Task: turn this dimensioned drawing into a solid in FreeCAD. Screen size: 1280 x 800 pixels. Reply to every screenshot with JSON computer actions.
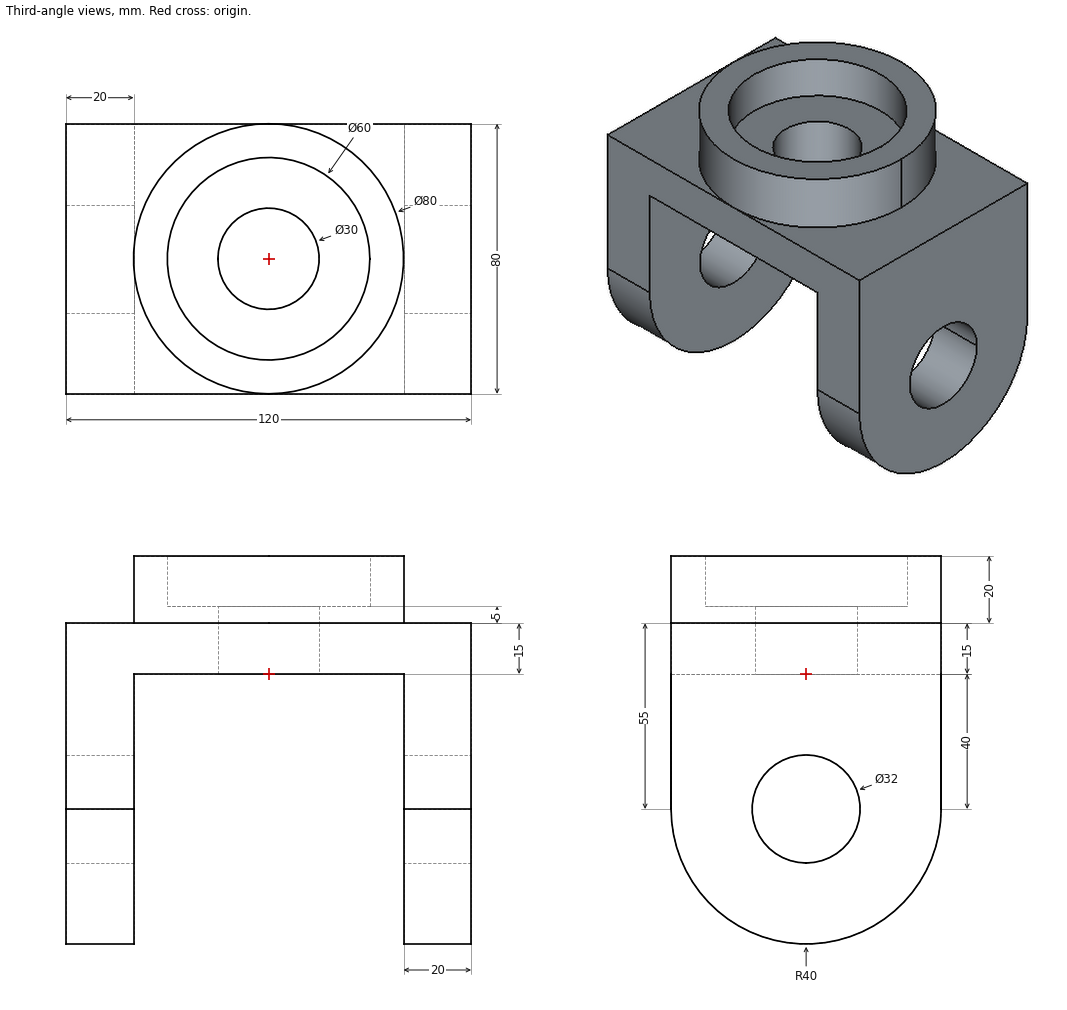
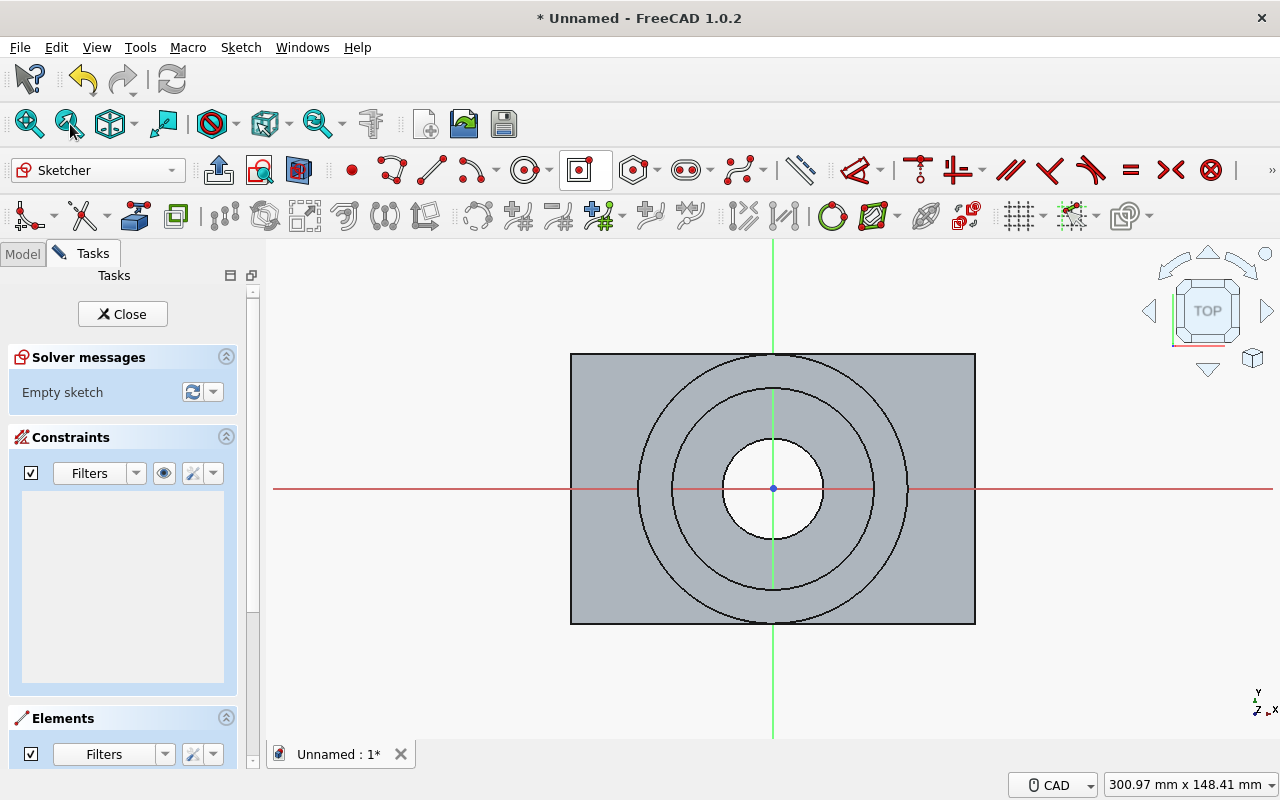
{"action": "left_click", "coordinate": [300, 170]}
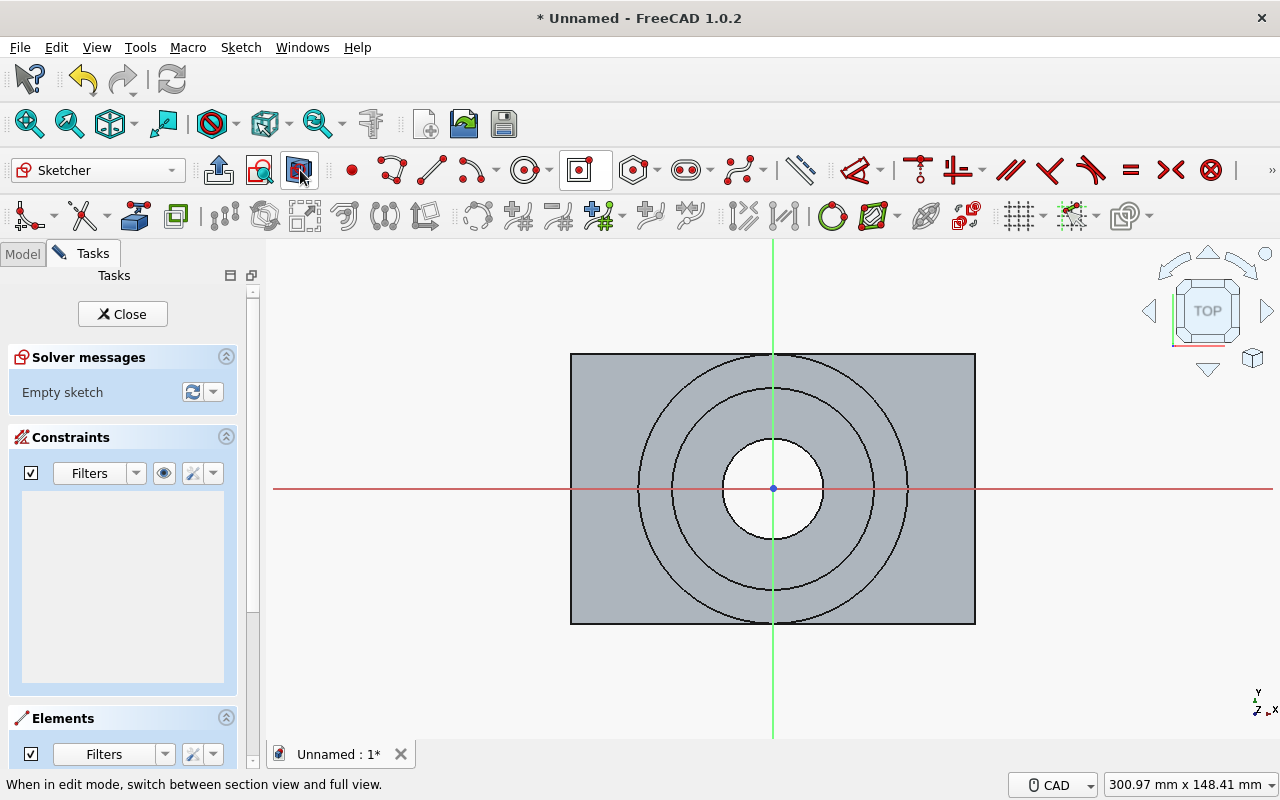
{"action": "scroll", "coordinate": [912, 489], "scroll_direction": "up", "scroll_amount": 2}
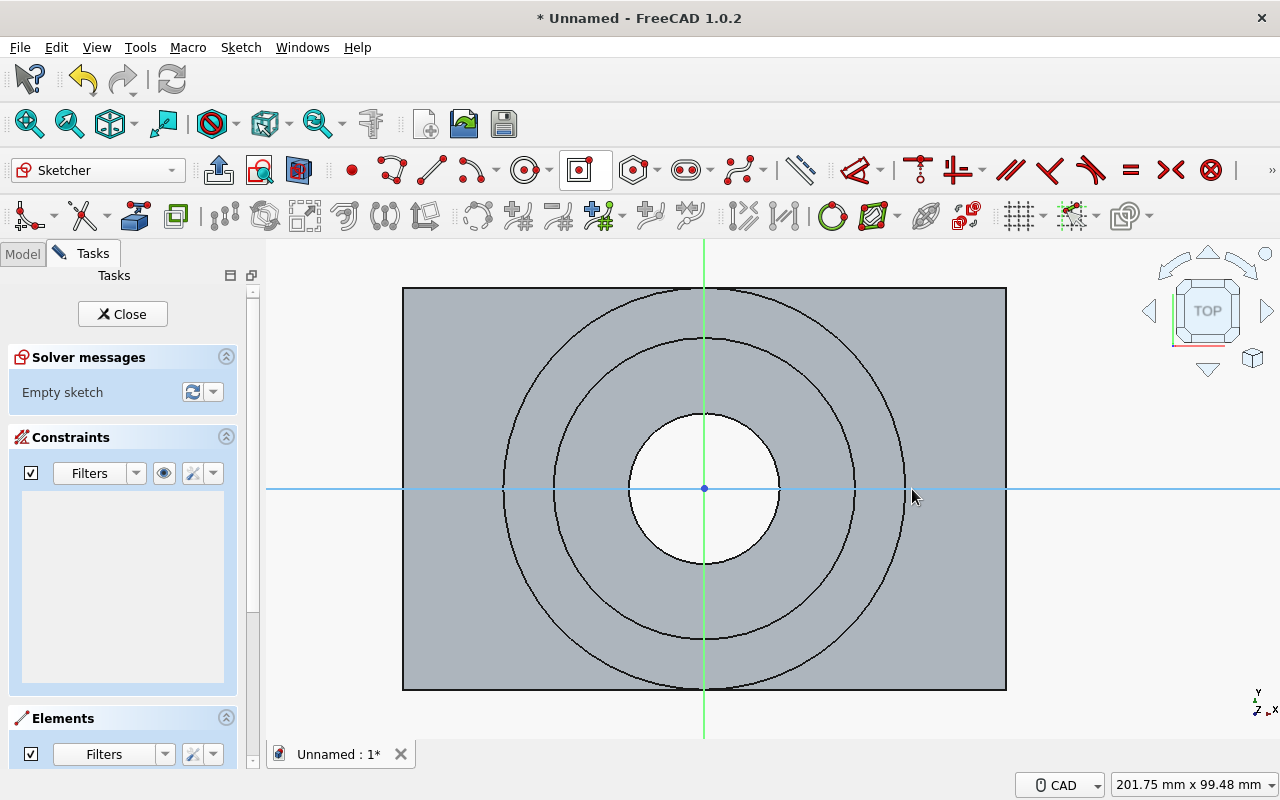
{"action": "key", "text": "g c"}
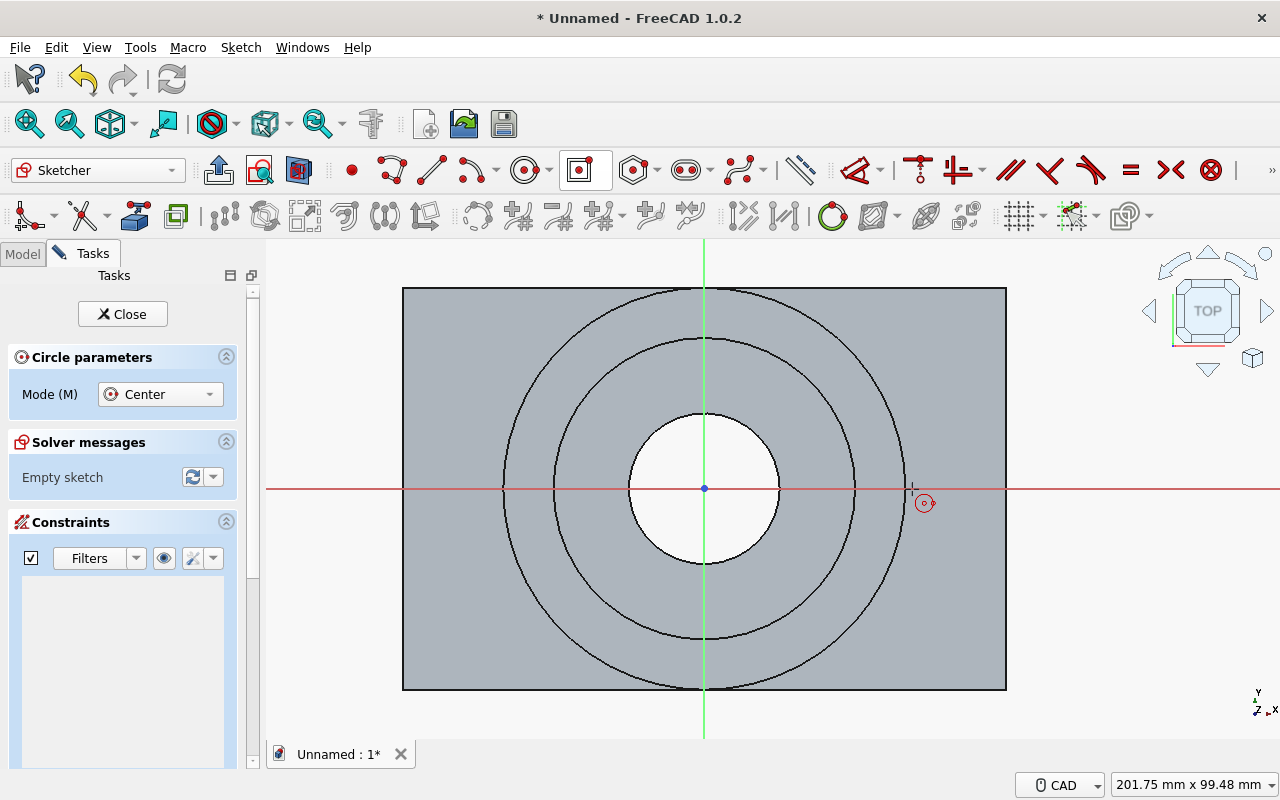
{"action": "left_click", "coordinate": [704, 489]}
{"action": "left_click", "coordinate": [811, 382]}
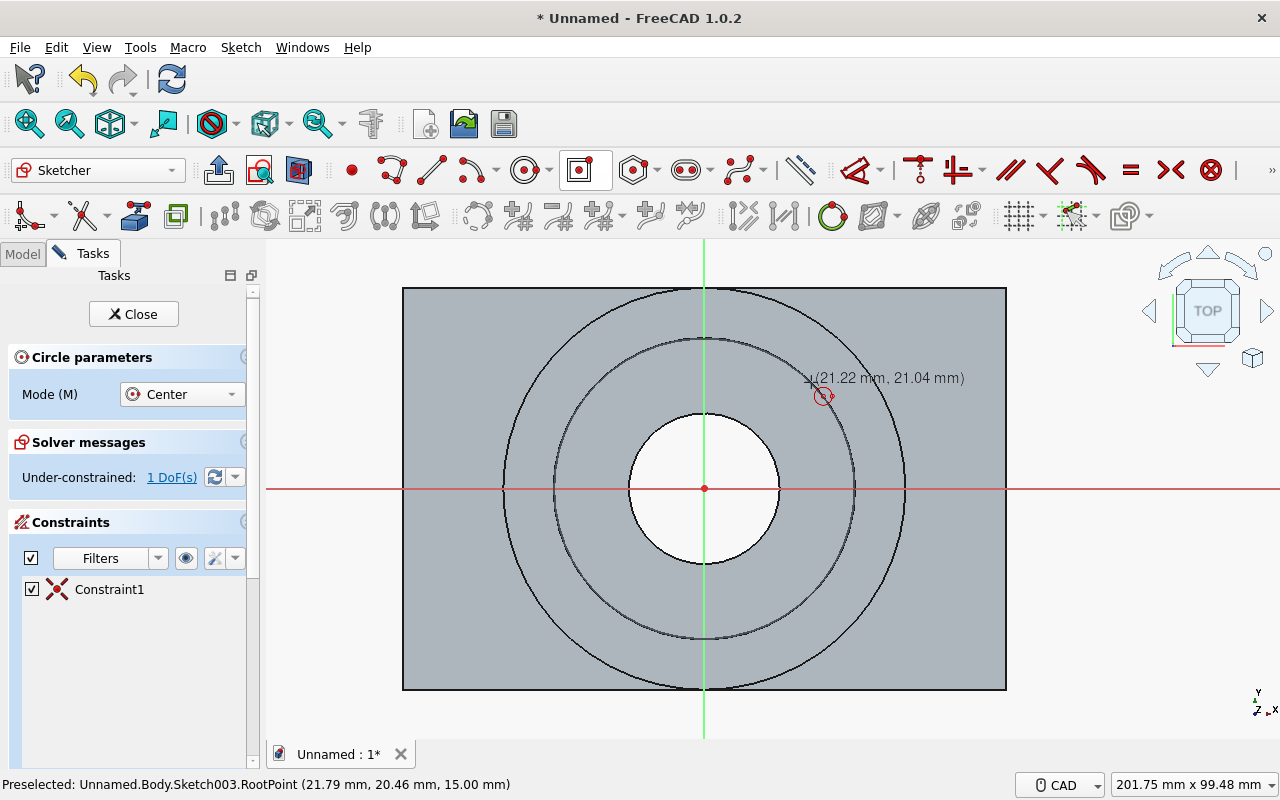
{"action": "left_click", "coordinate": [704, 489]}
{"action": "left_click", "coordinate": [758, 435]}
{"action": "key", "text": "Escape"}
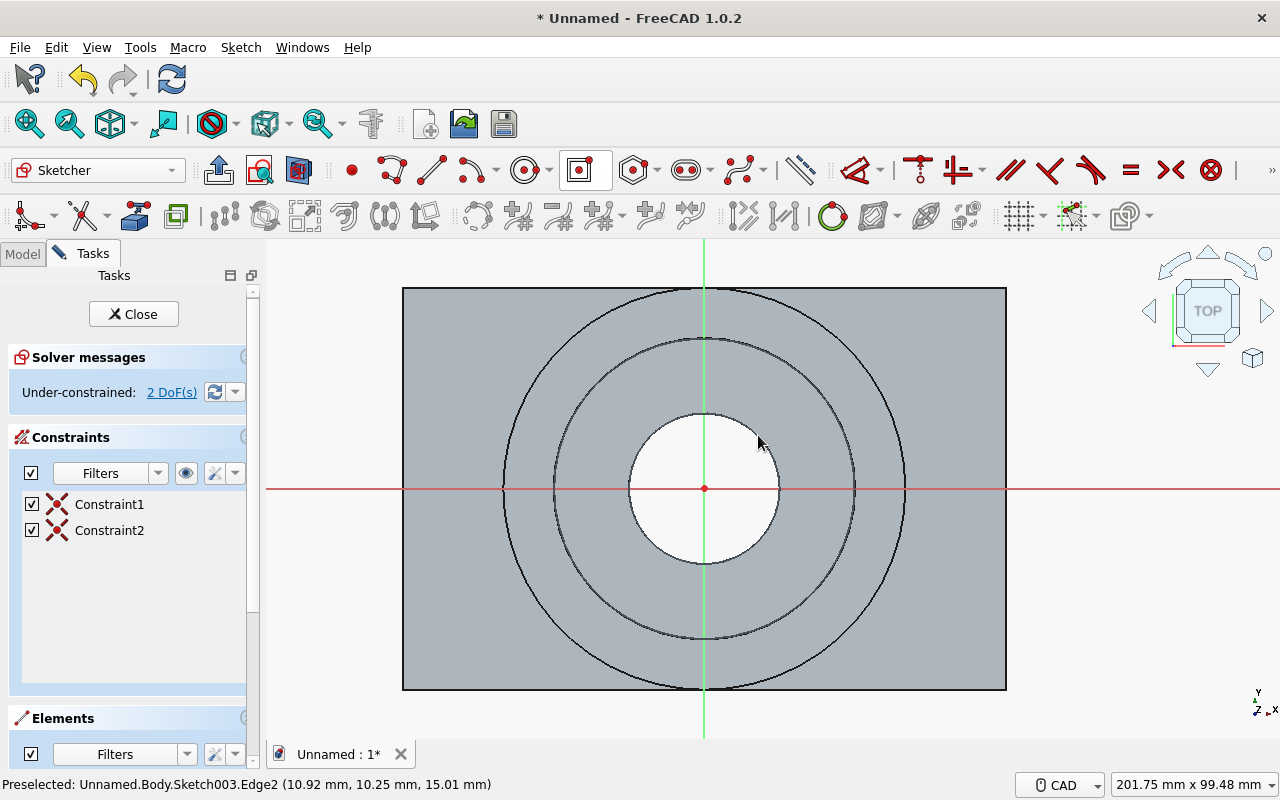
{"action": "left_click", "coordinate": [856, 170]}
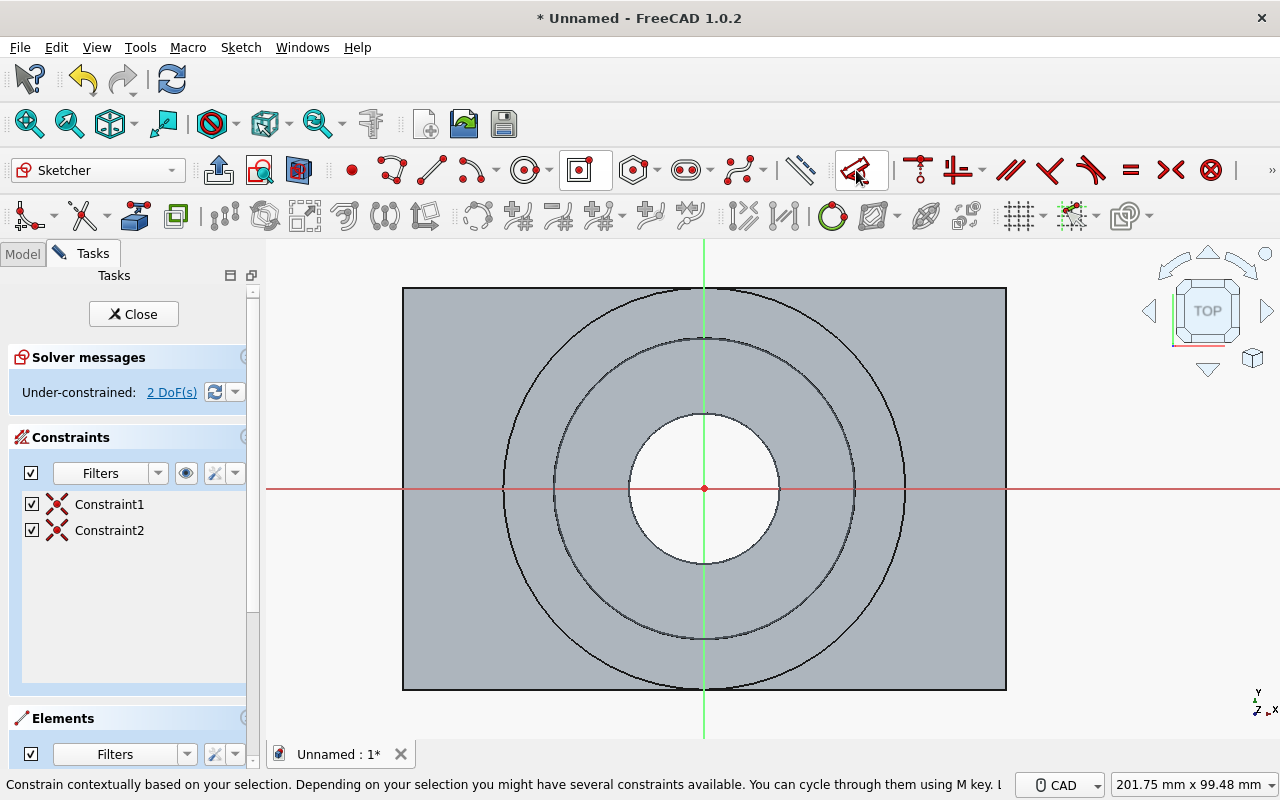
{"action": "left_click", "coordinate": [810, 382]}
{"action": "left_click", "coordinate": [833, 359]}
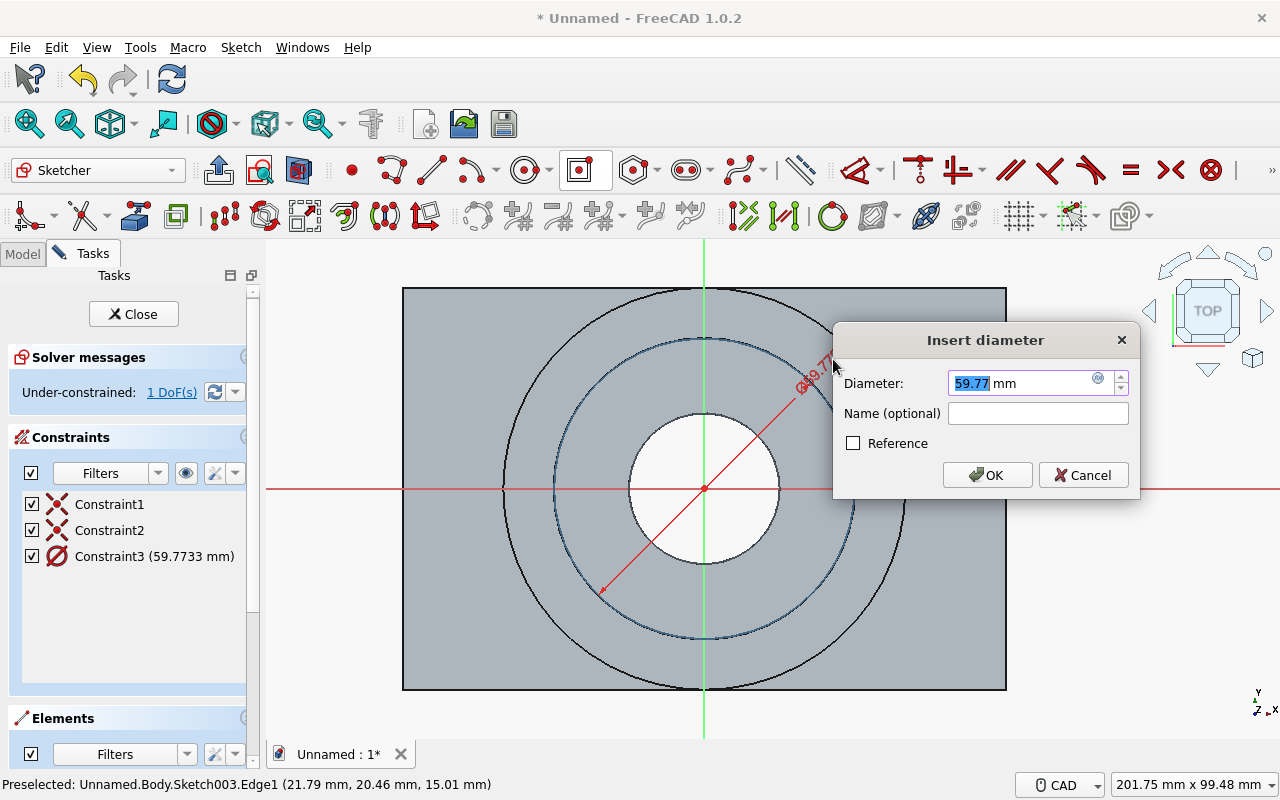
{"action": "type", "text": "60"}
{"action": "key", "text": "Return"}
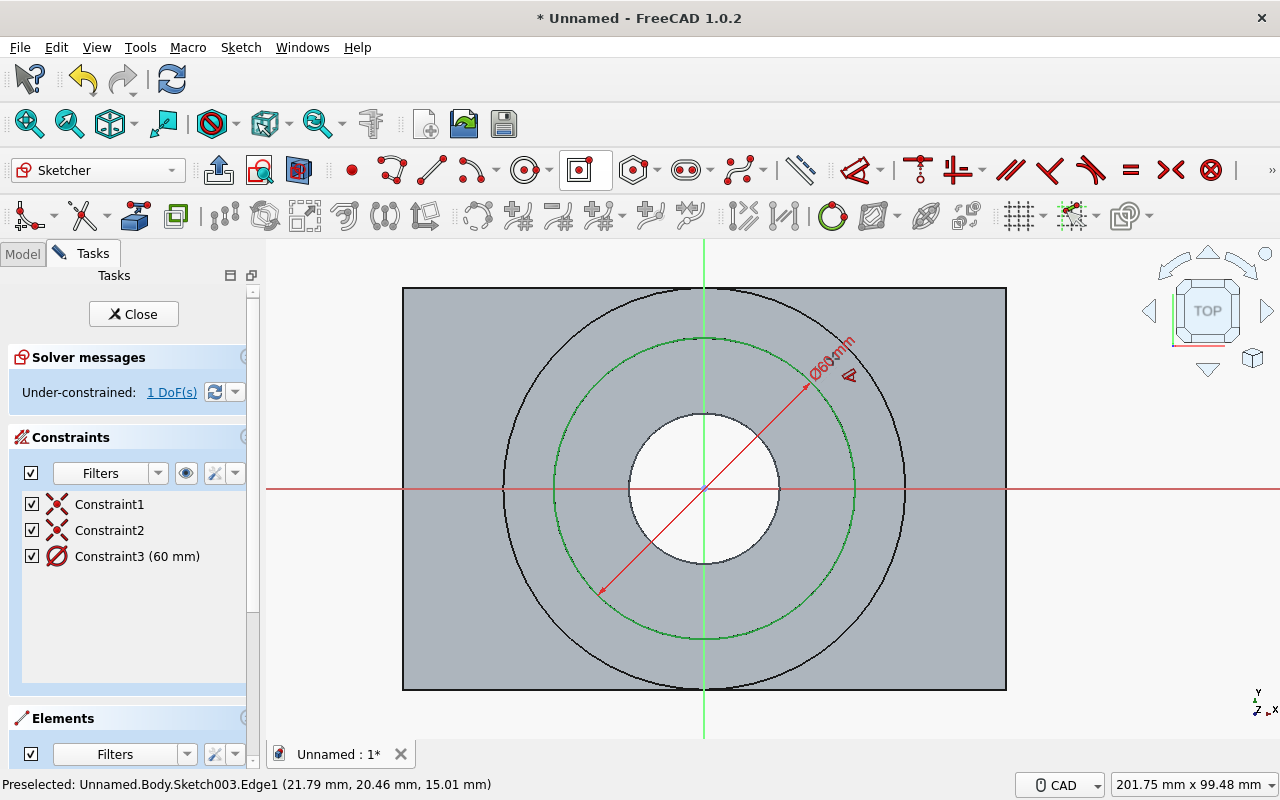
{"action": "left_click", "coordinate": [757, 435]}
{"action": "left_click", "coordinate": [779, 412]}